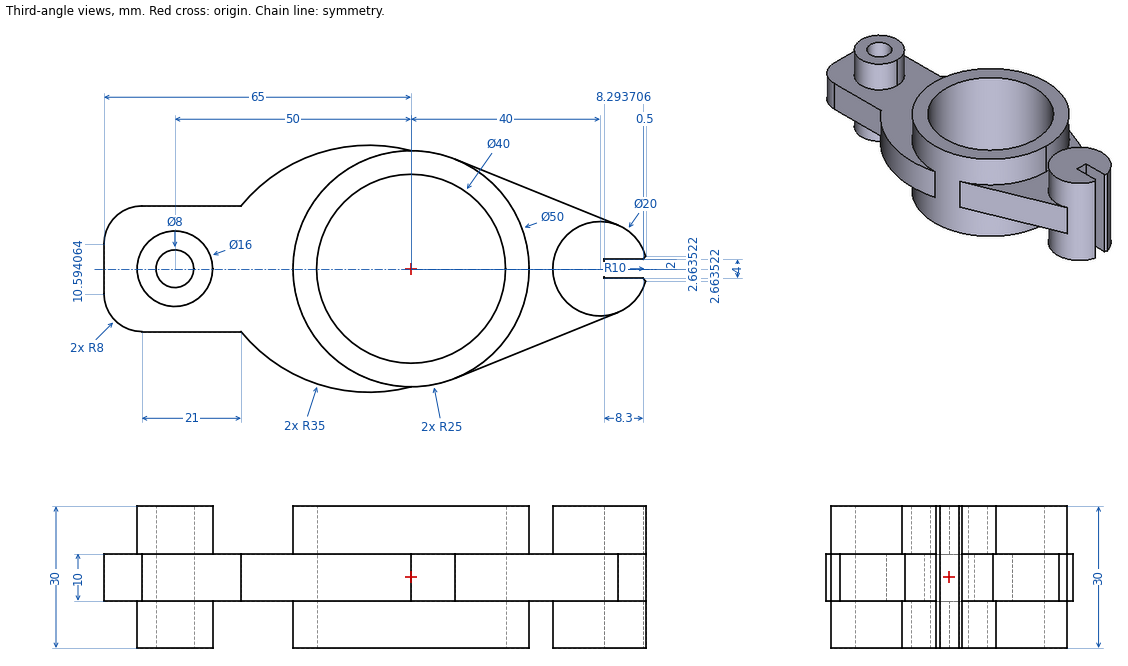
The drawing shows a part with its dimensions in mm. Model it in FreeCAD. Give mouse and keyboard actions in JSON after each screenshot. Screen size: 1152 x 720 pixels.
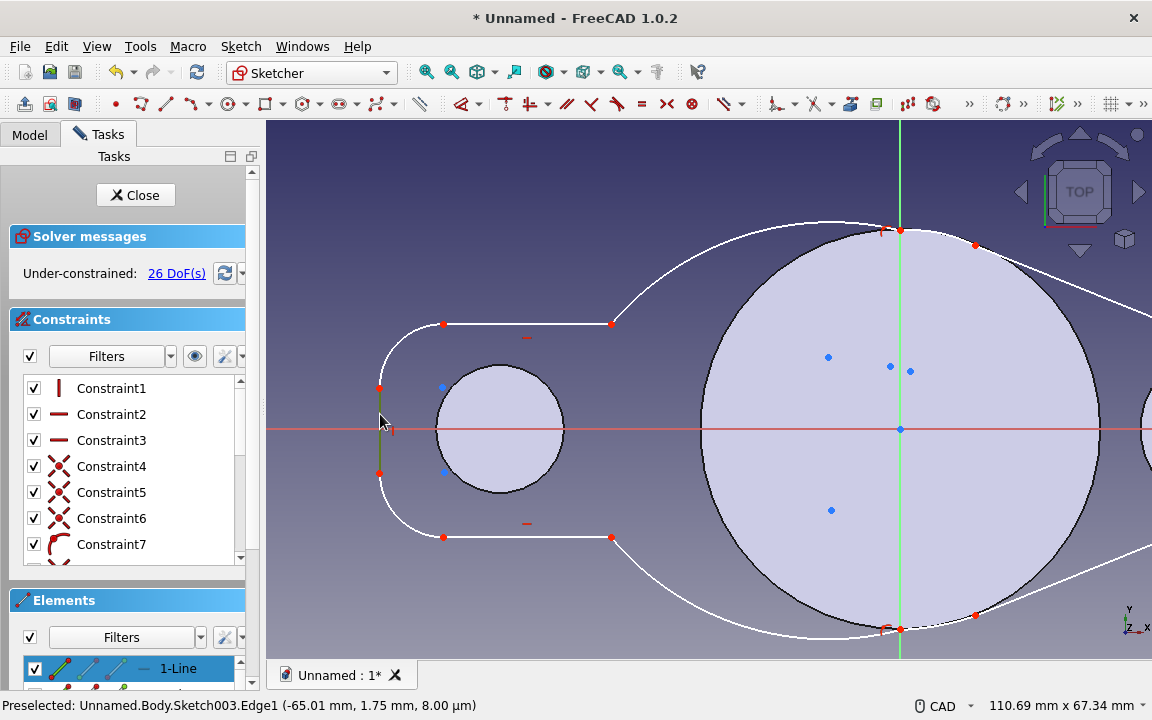
{"action": "left_click", "coordinate": [387, 502]}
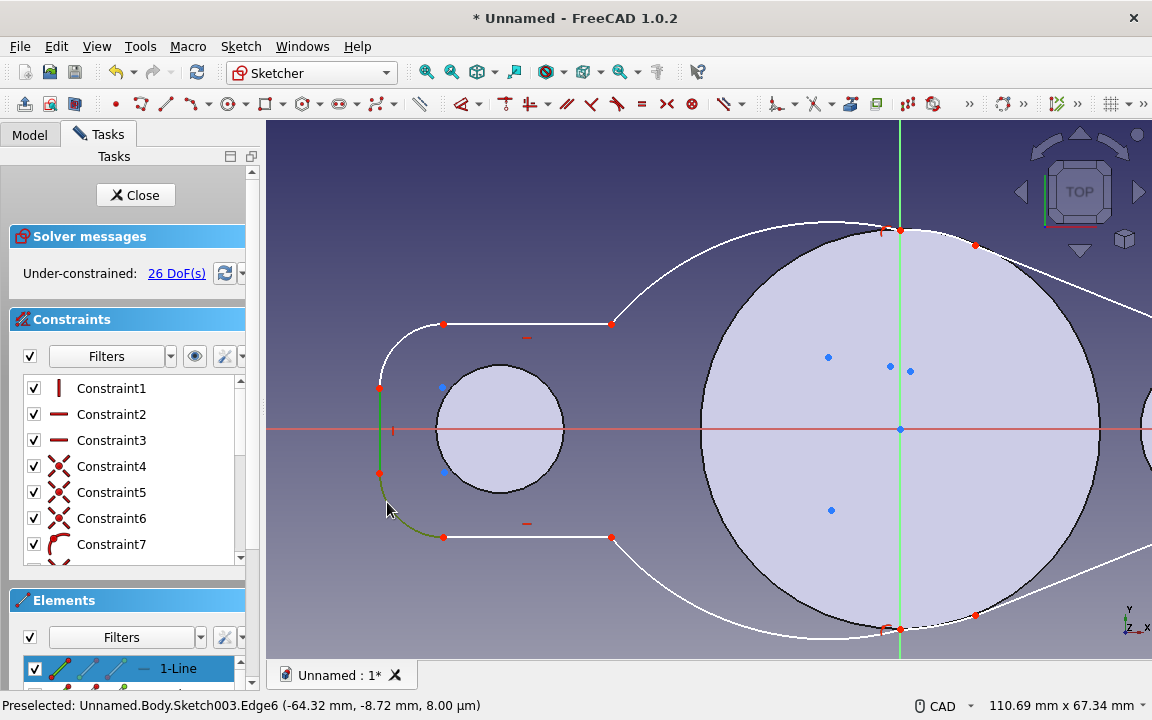
{"action": "left_click", "coordinate": [617, 104]}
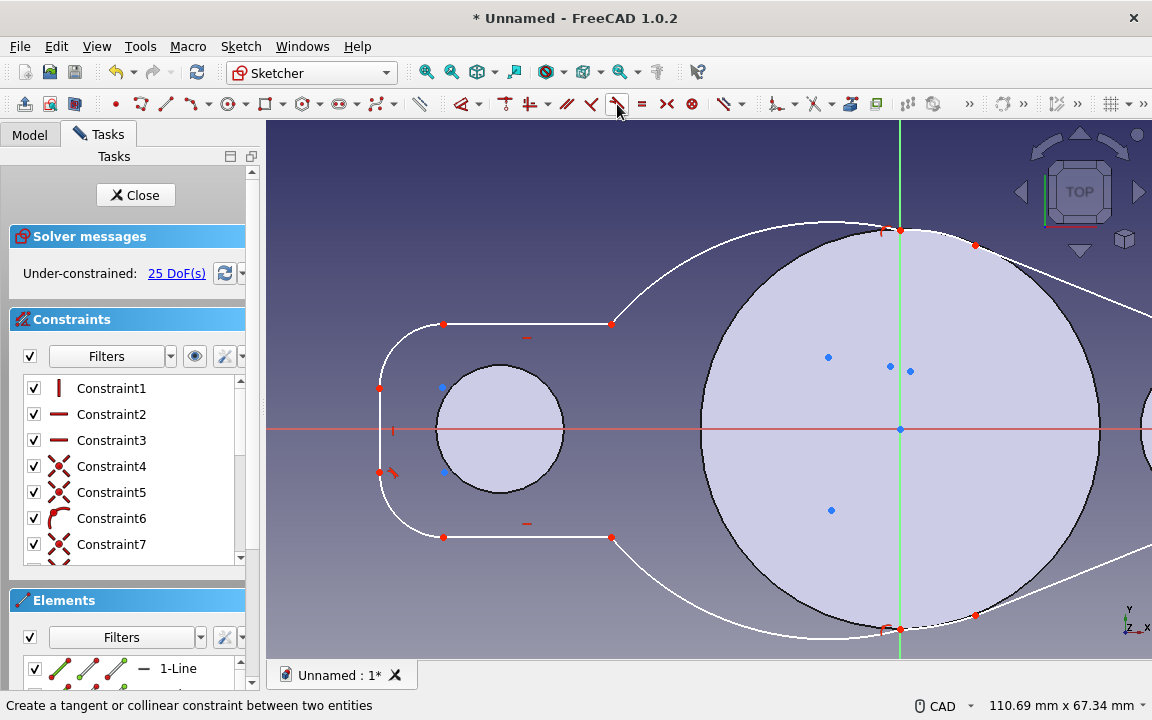
{"action": "left_click", "coordinate": [380, 413]}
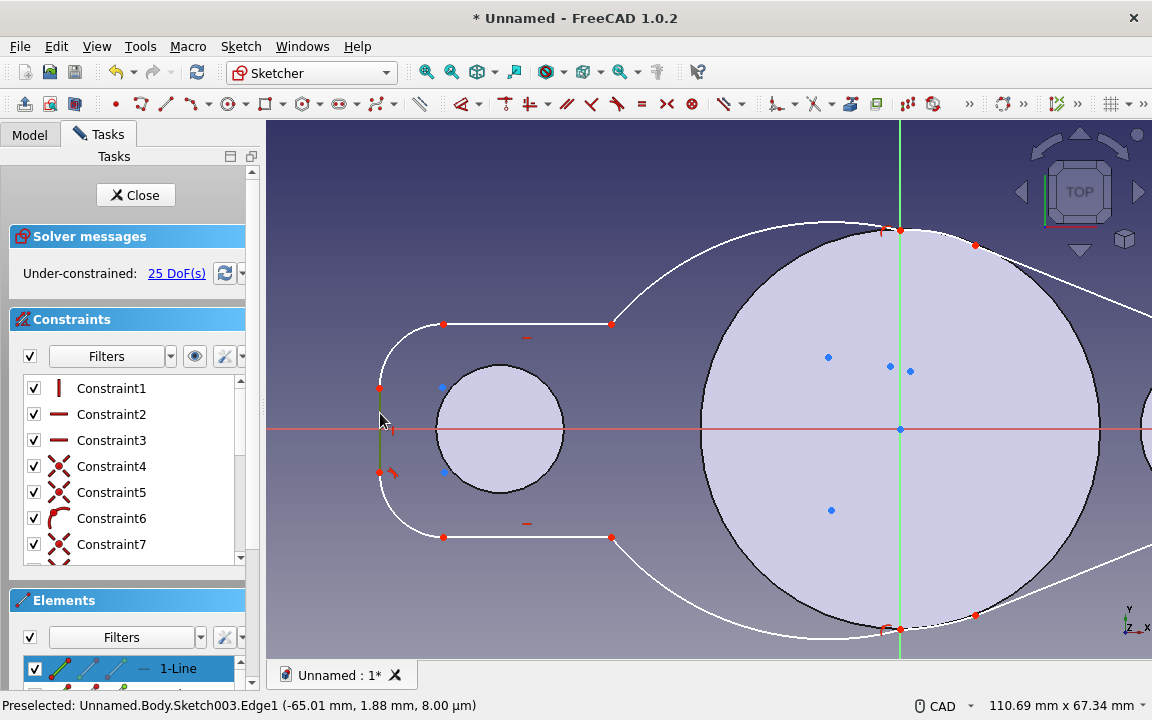
{"action": "left_click", "coordinate": [415, 331]}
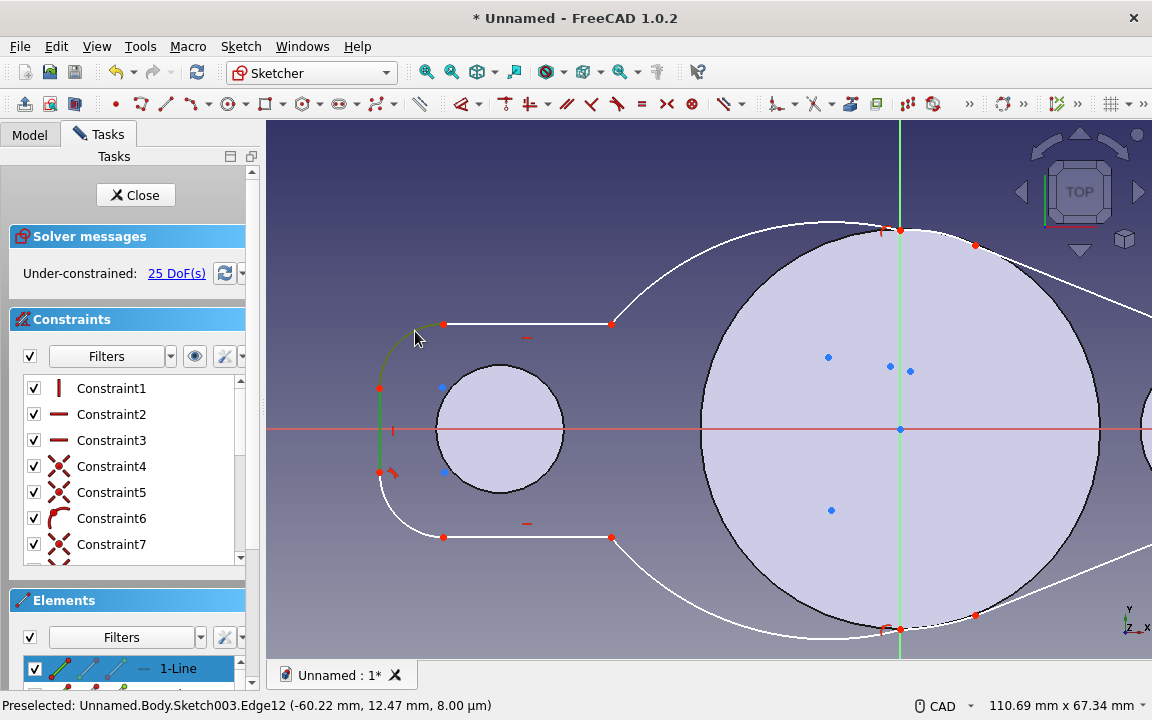
{"action": "left_click", "coordinate": [617, 104]}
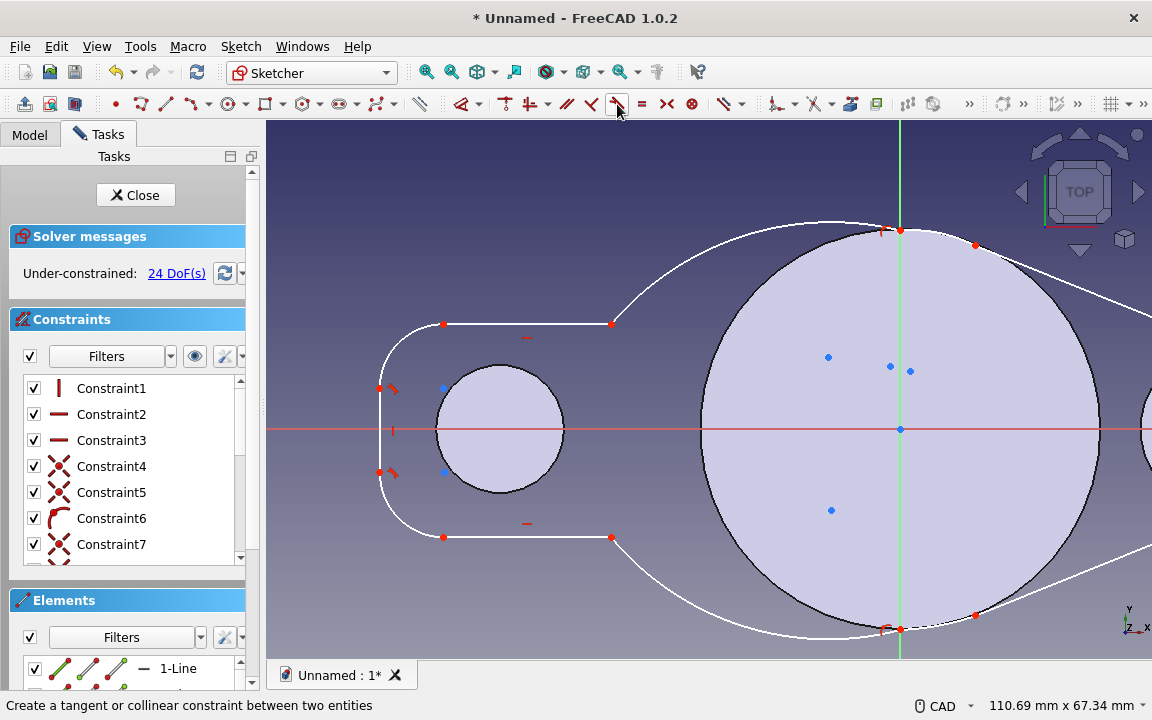
{"action": "left_click", "coordinate": [494, 537]}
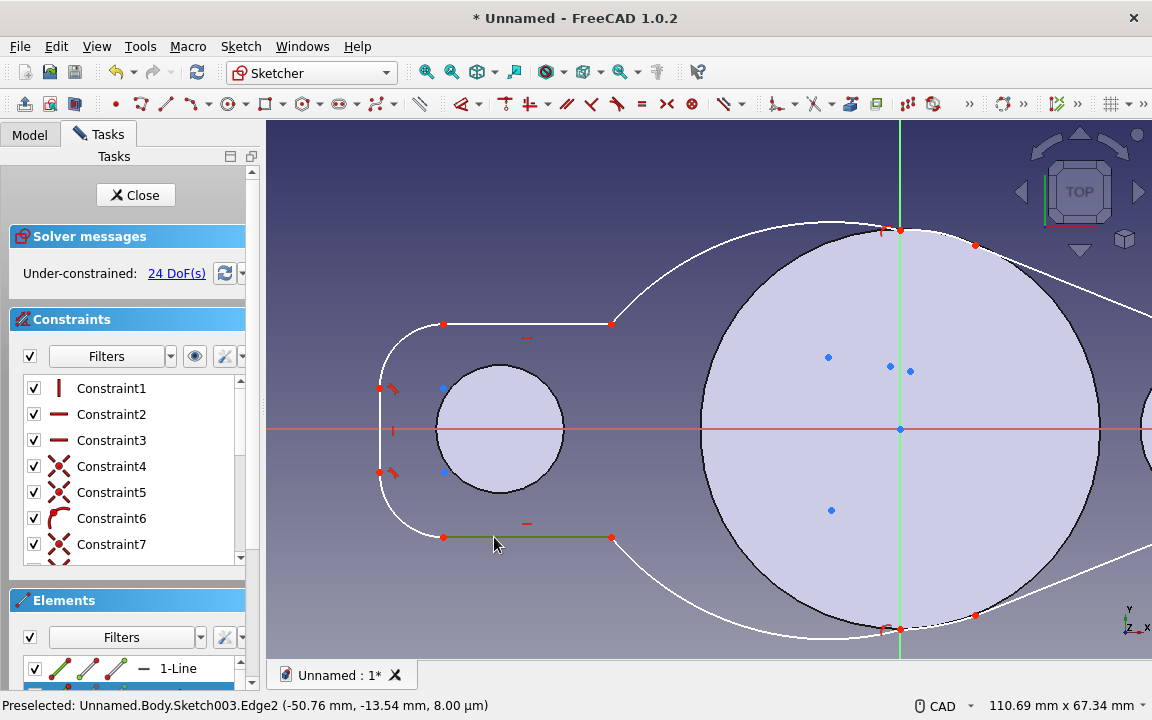
{"action": "left_click", "coordinate": [387, 502]}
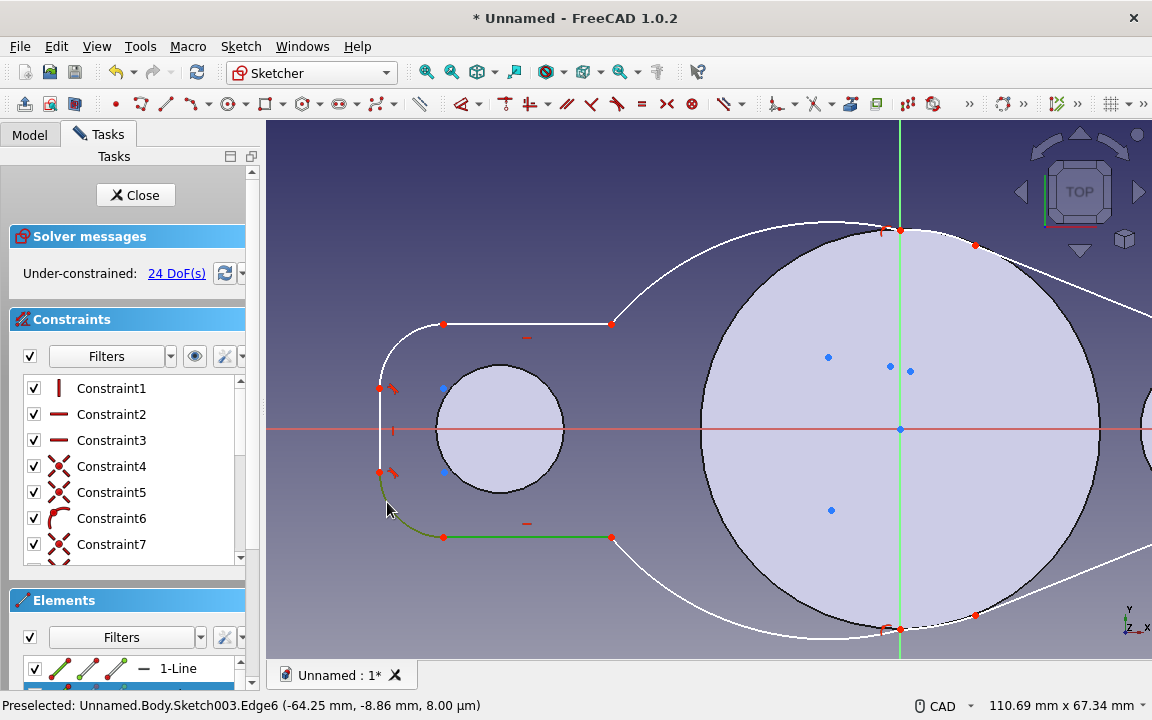
{"action": "left_click", "coordinate": [617, 104]}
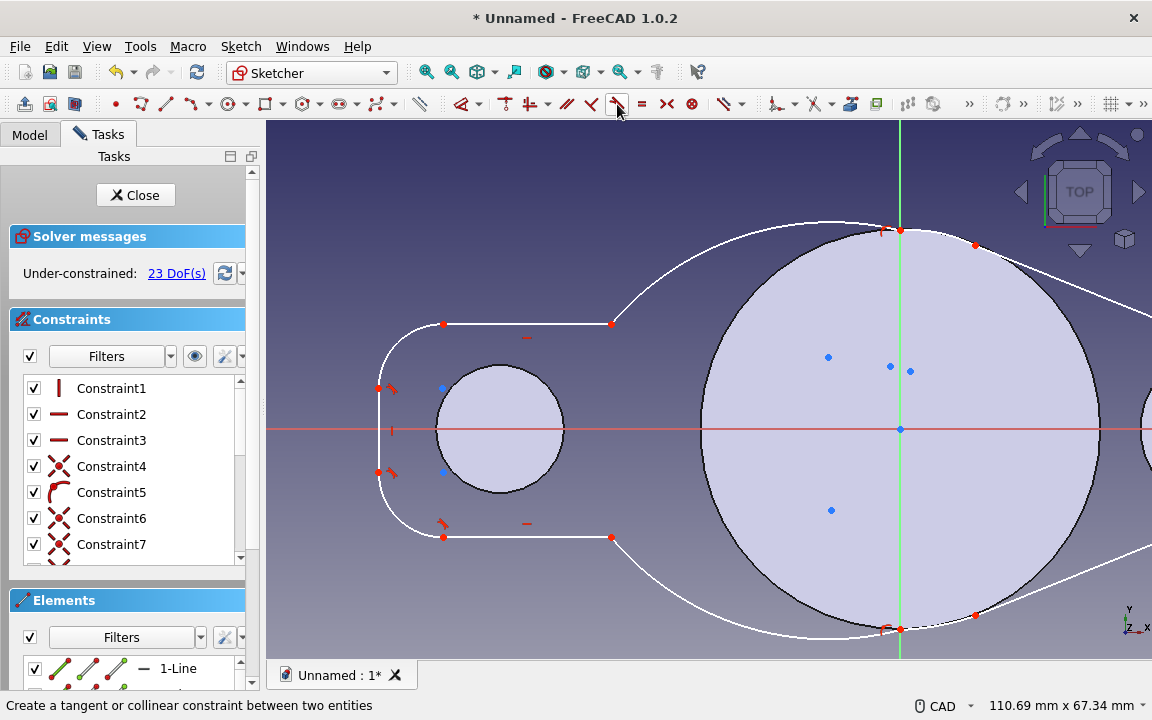
{"action": "scroll", "coordinate": [398, 341], "scroll_direction": "down", "scroll_amount": 3}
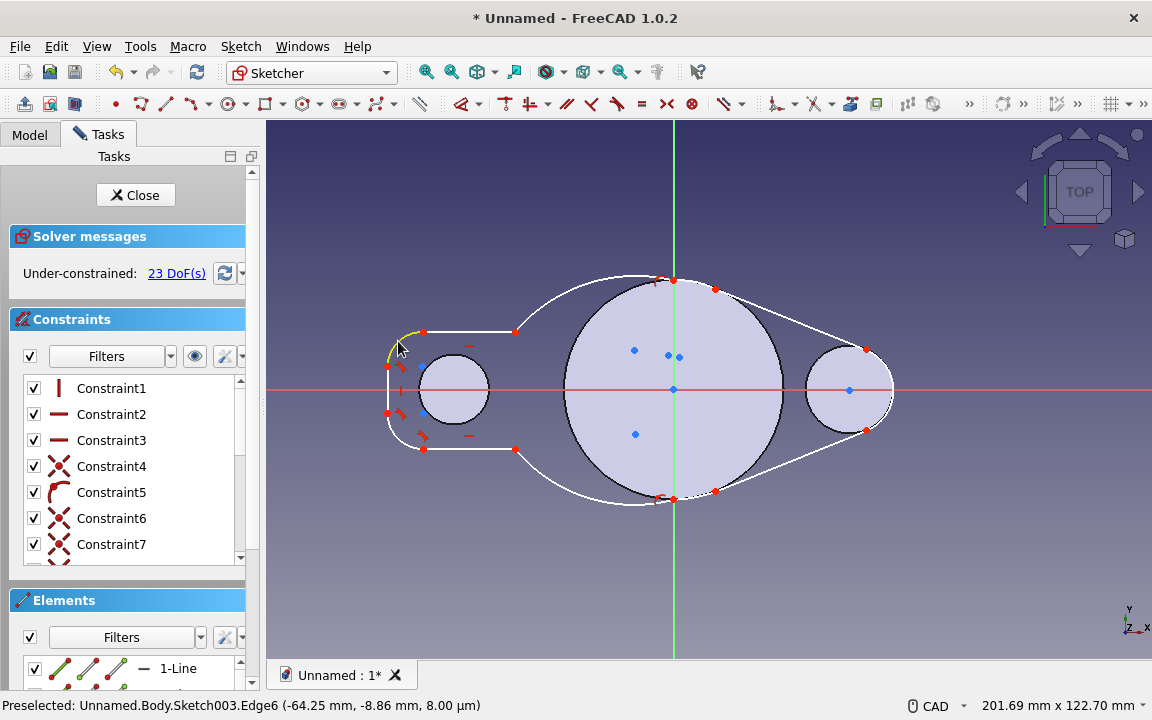
{"action": "left_click", "coordinate": [760, 474]}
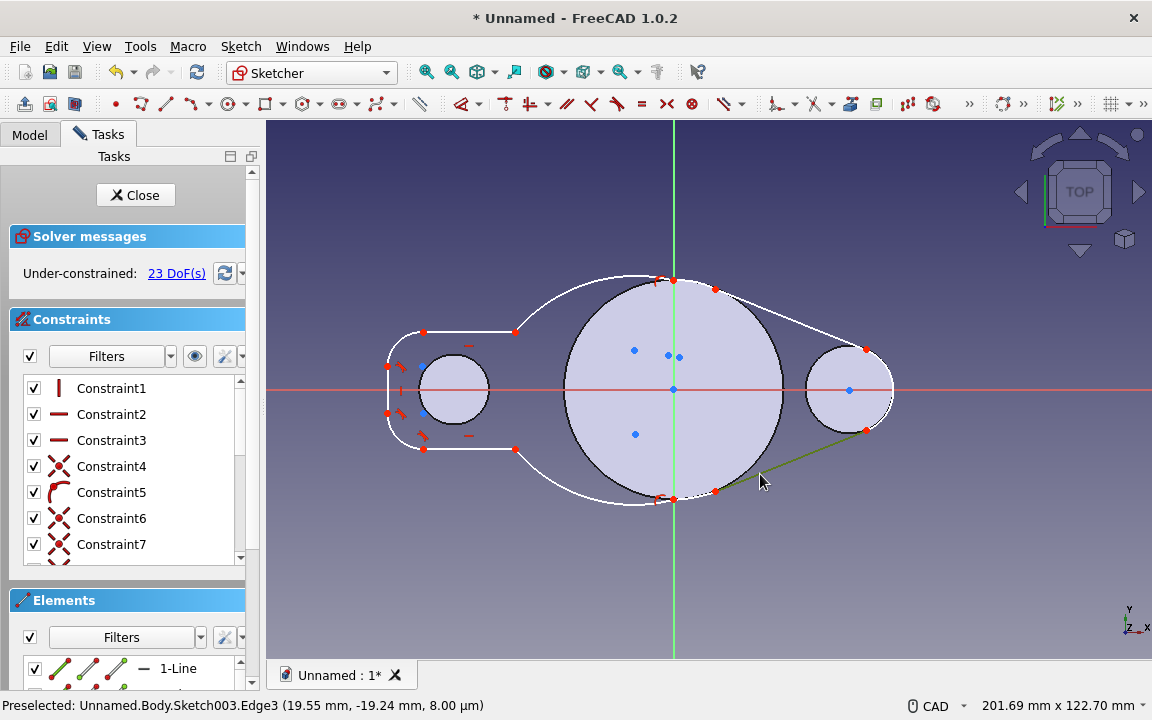
{"action": "left_click", "coordinate": [686, 499]}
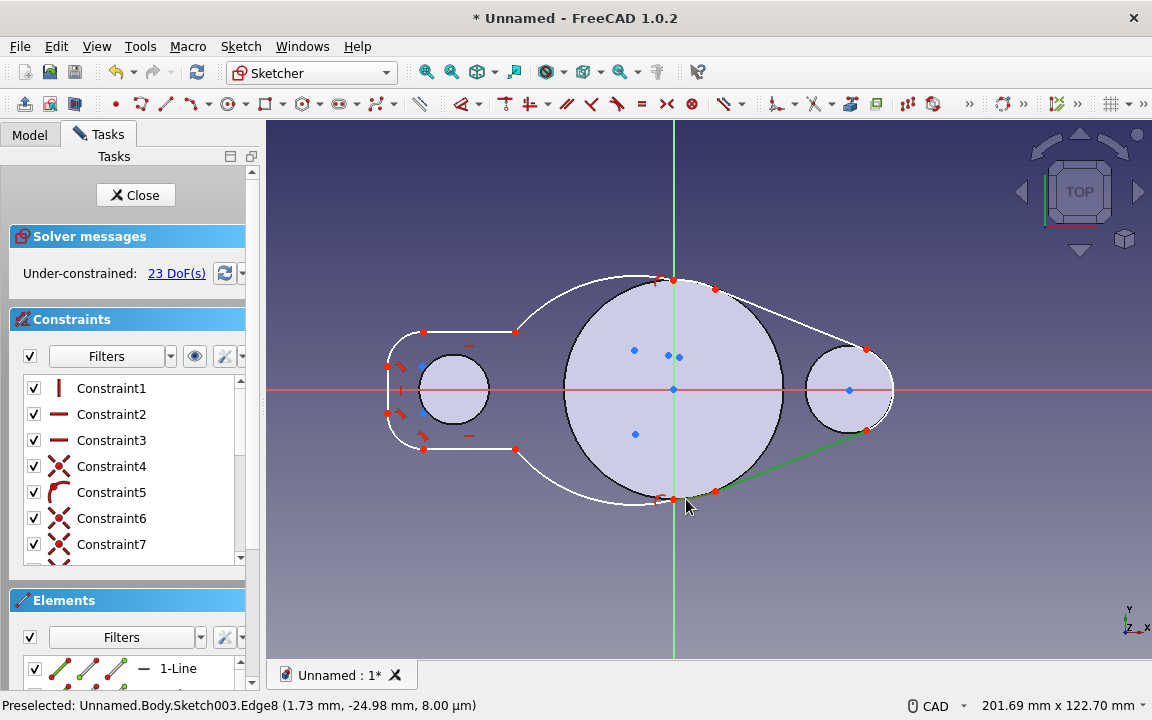
{"action": "left_click", "coordinate": [617, 104]}